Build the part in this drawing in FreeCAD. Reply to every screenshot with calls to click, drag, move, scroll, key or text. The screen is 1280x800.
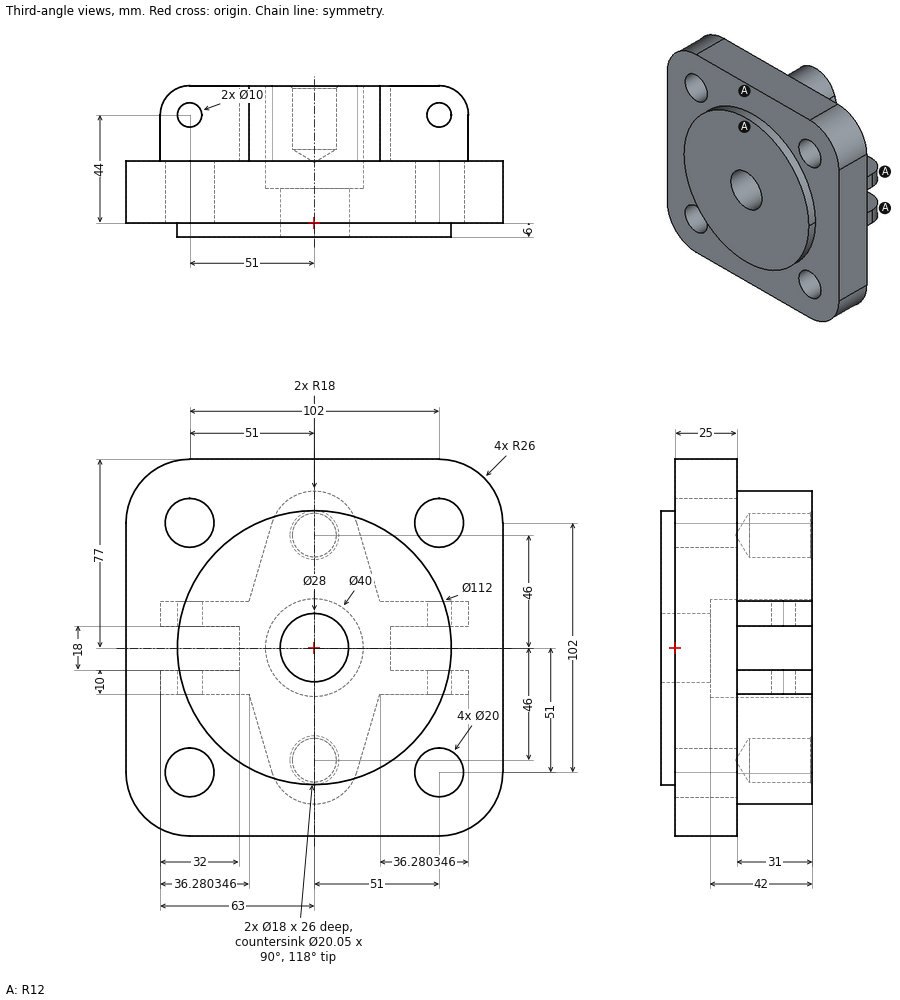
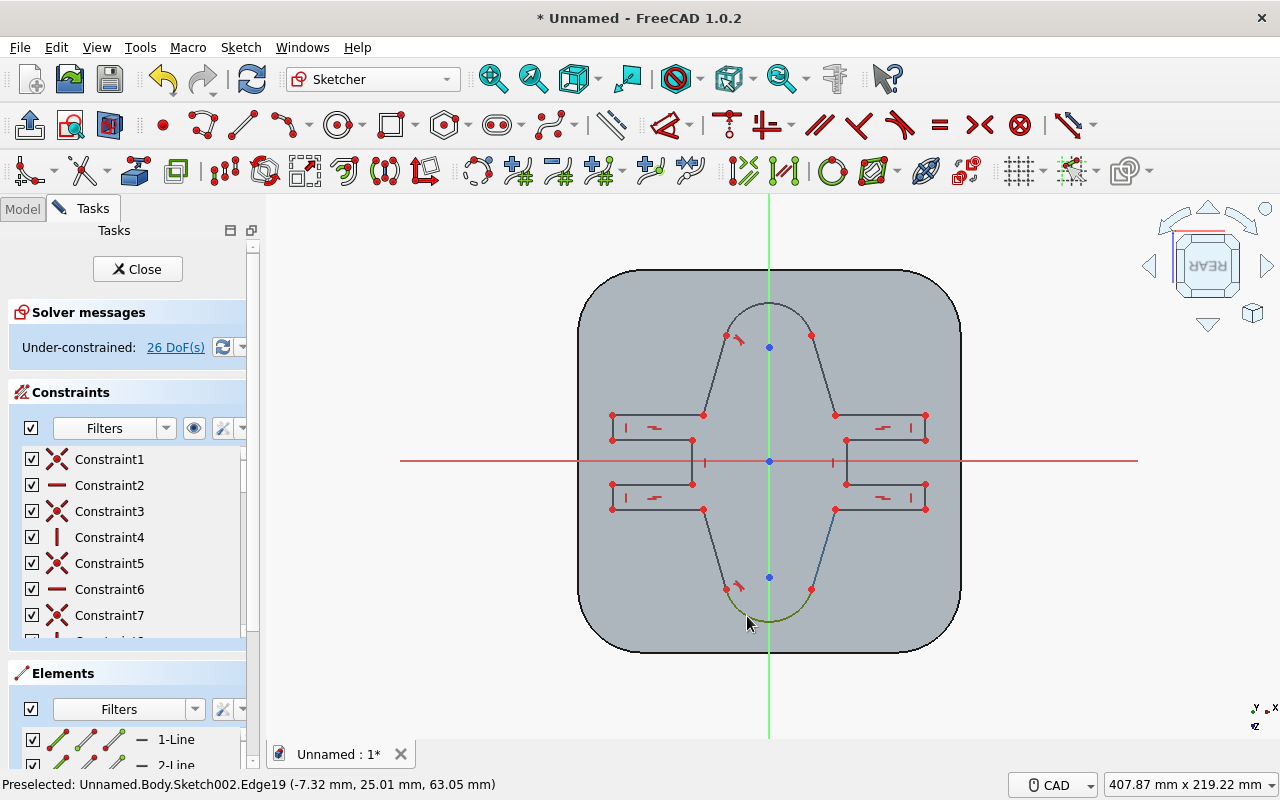
click(900, 126)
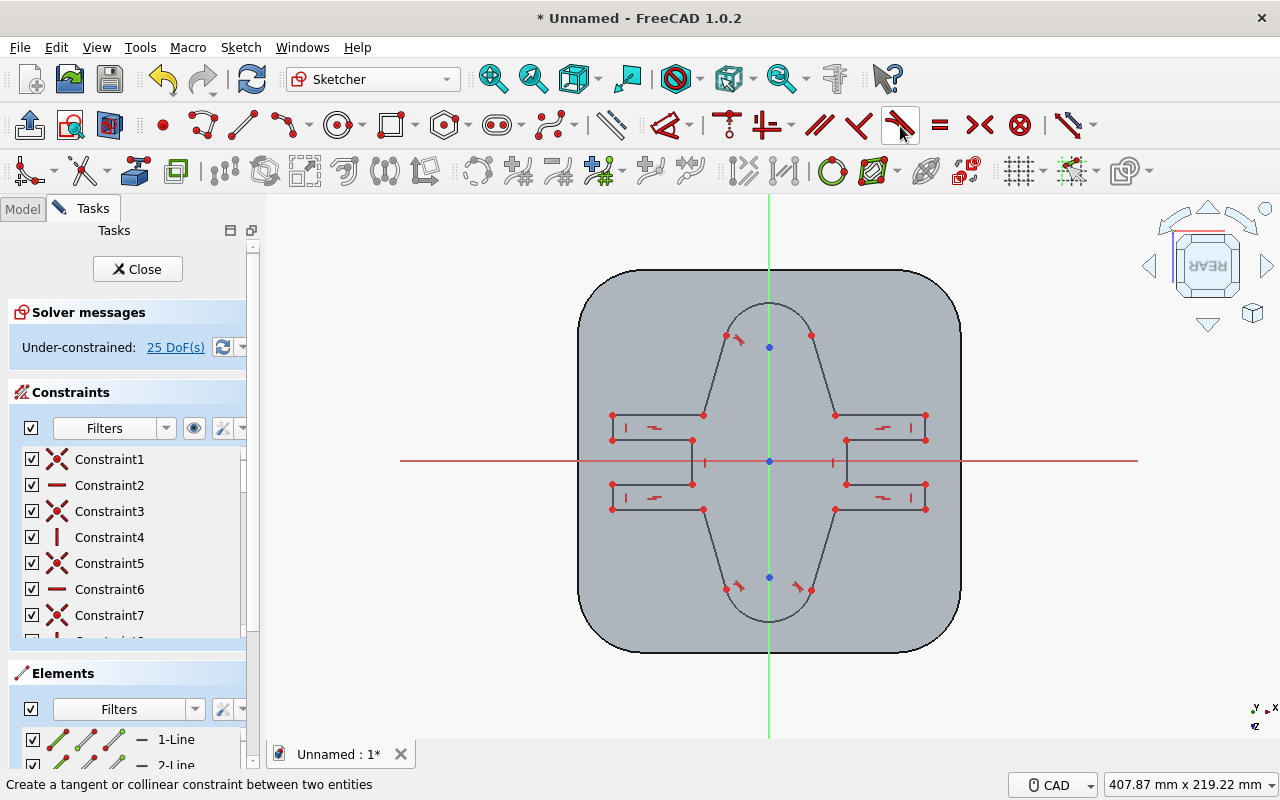
click(829, 391)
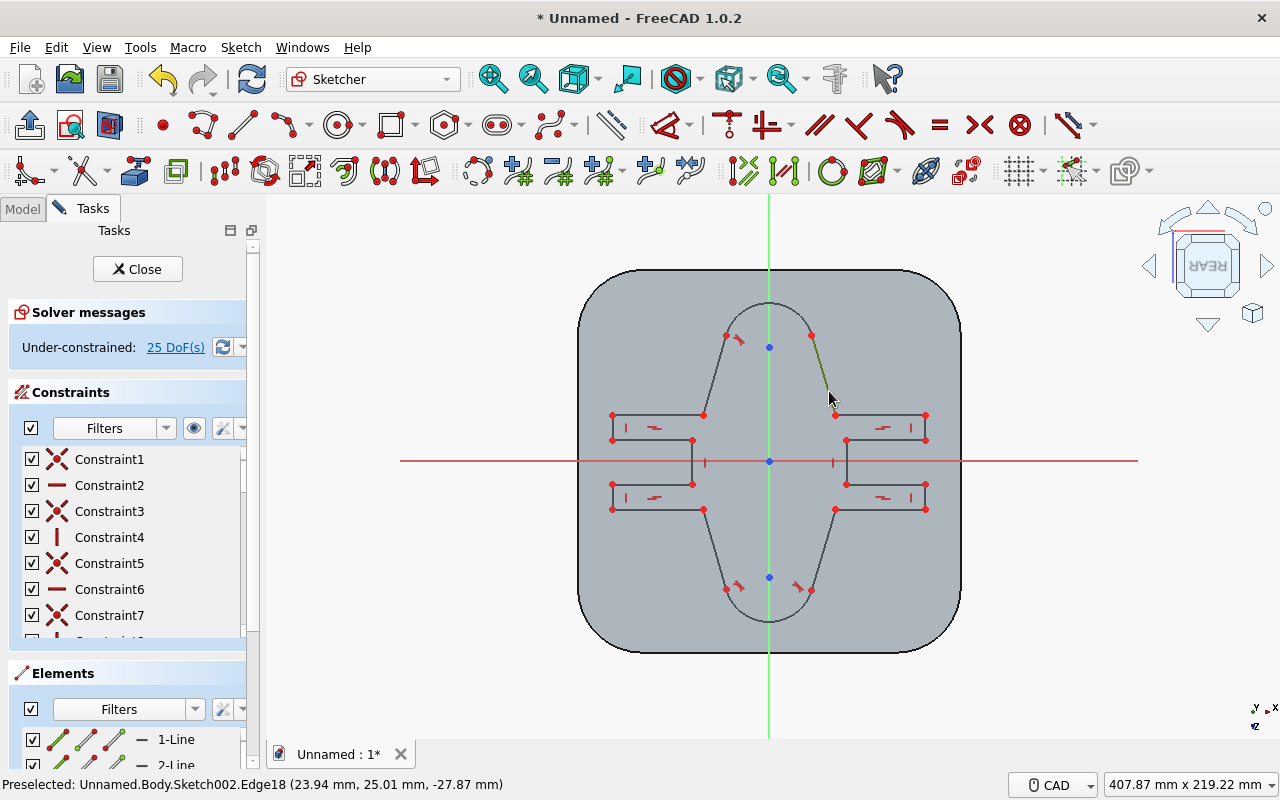
click(791, 309)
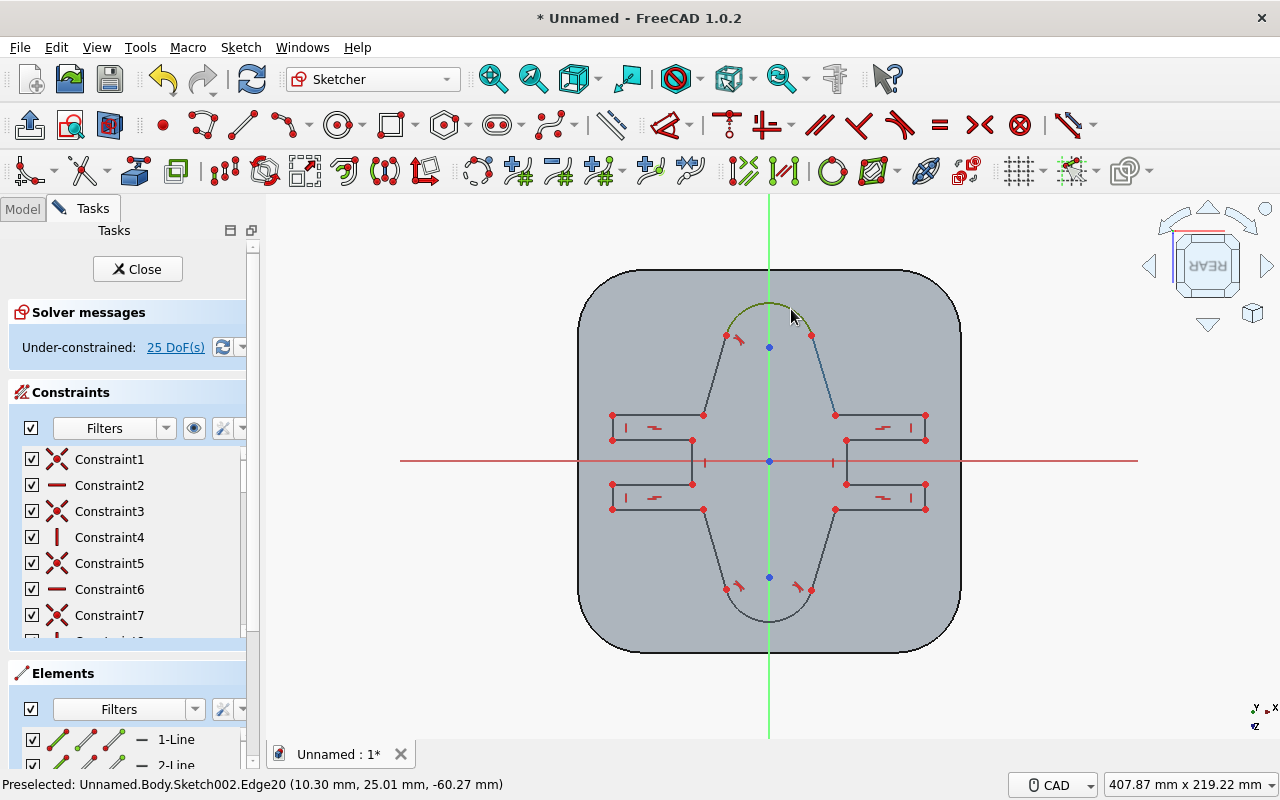
key(t)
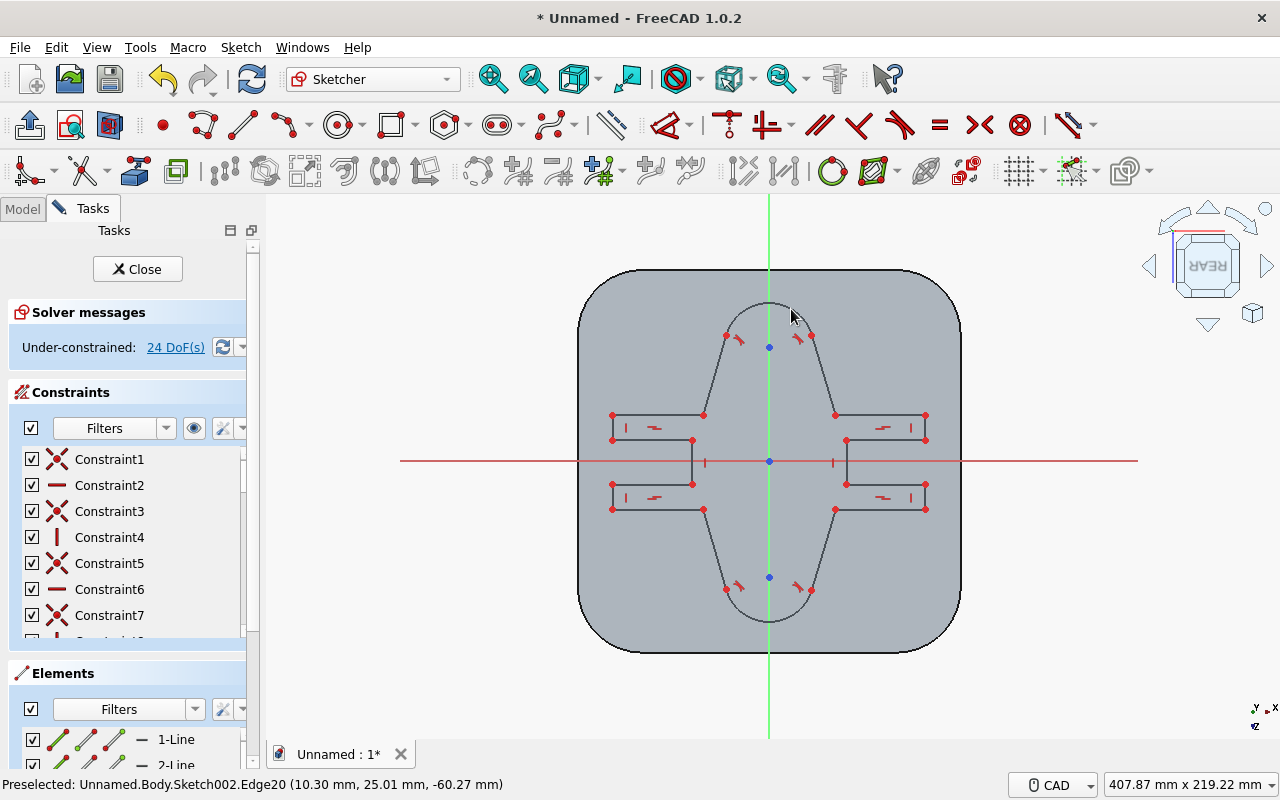
click(747, 616)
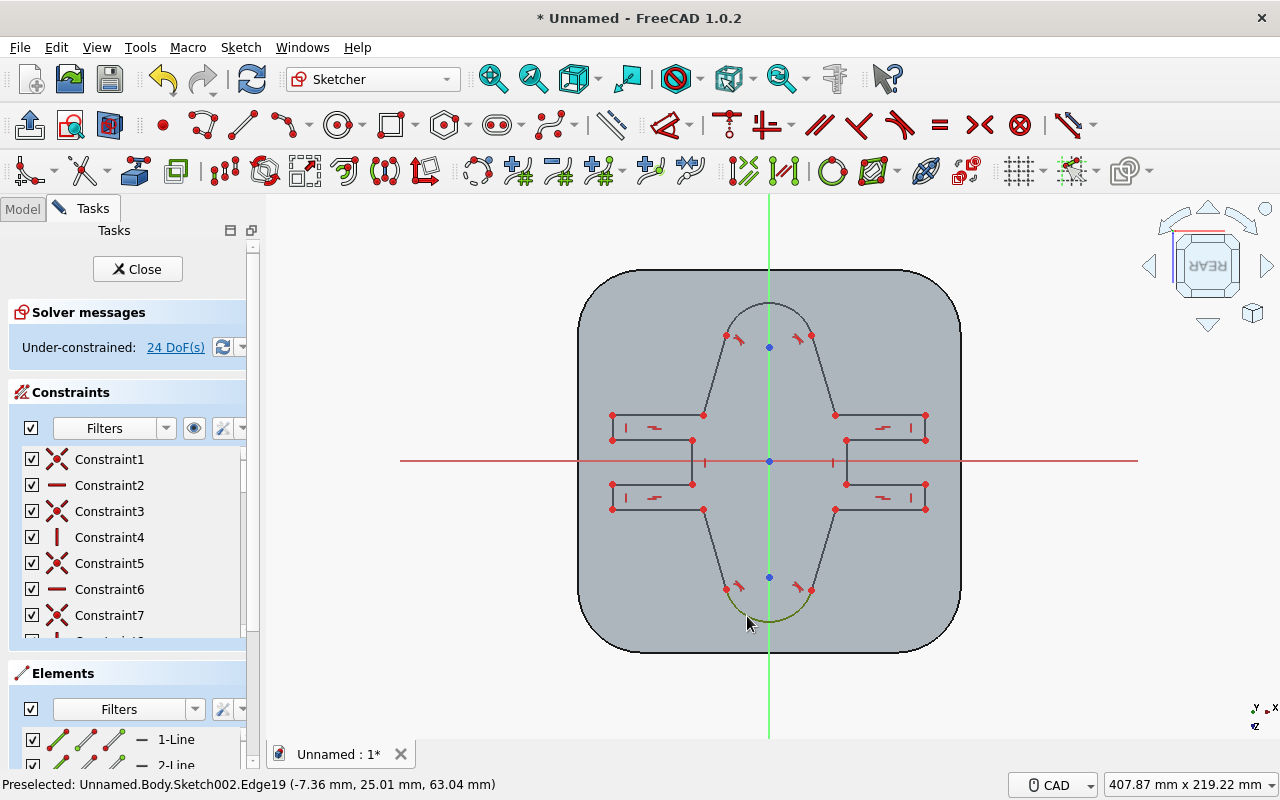
click(791, 309)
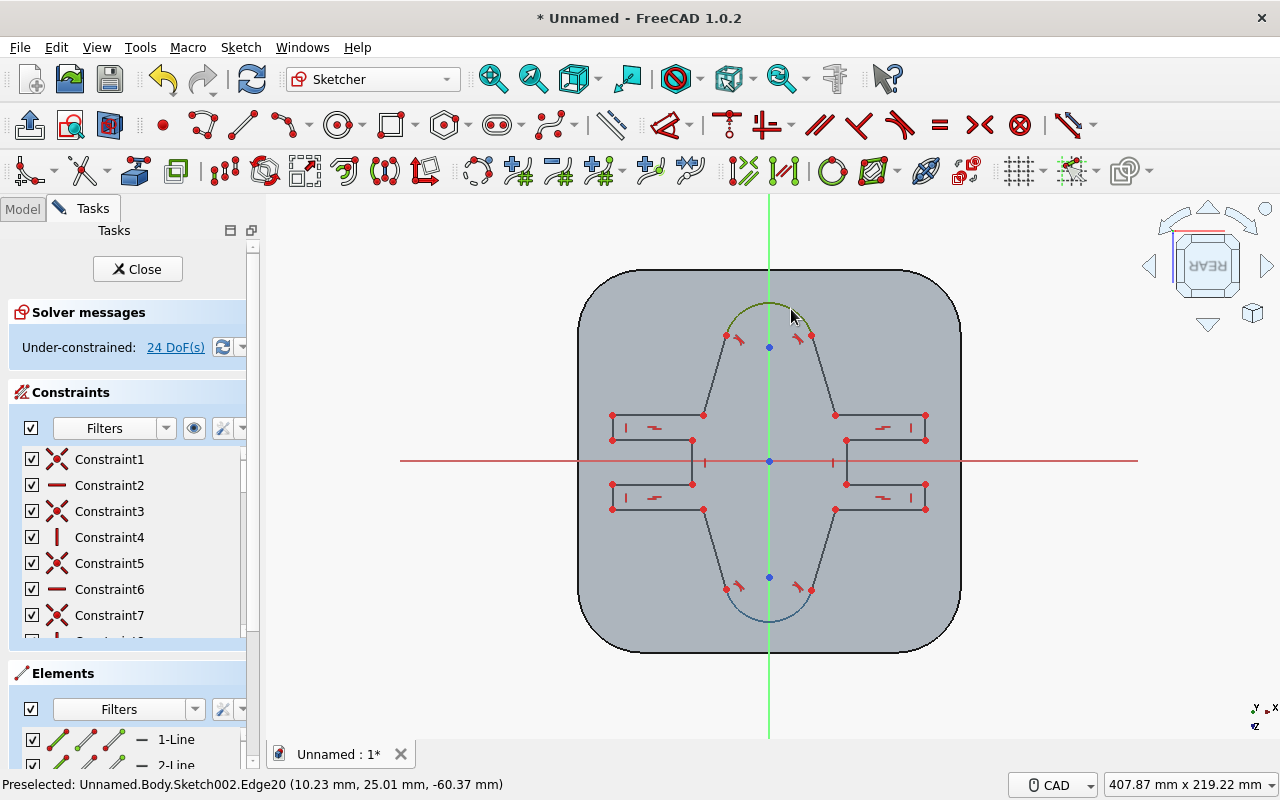
key(e)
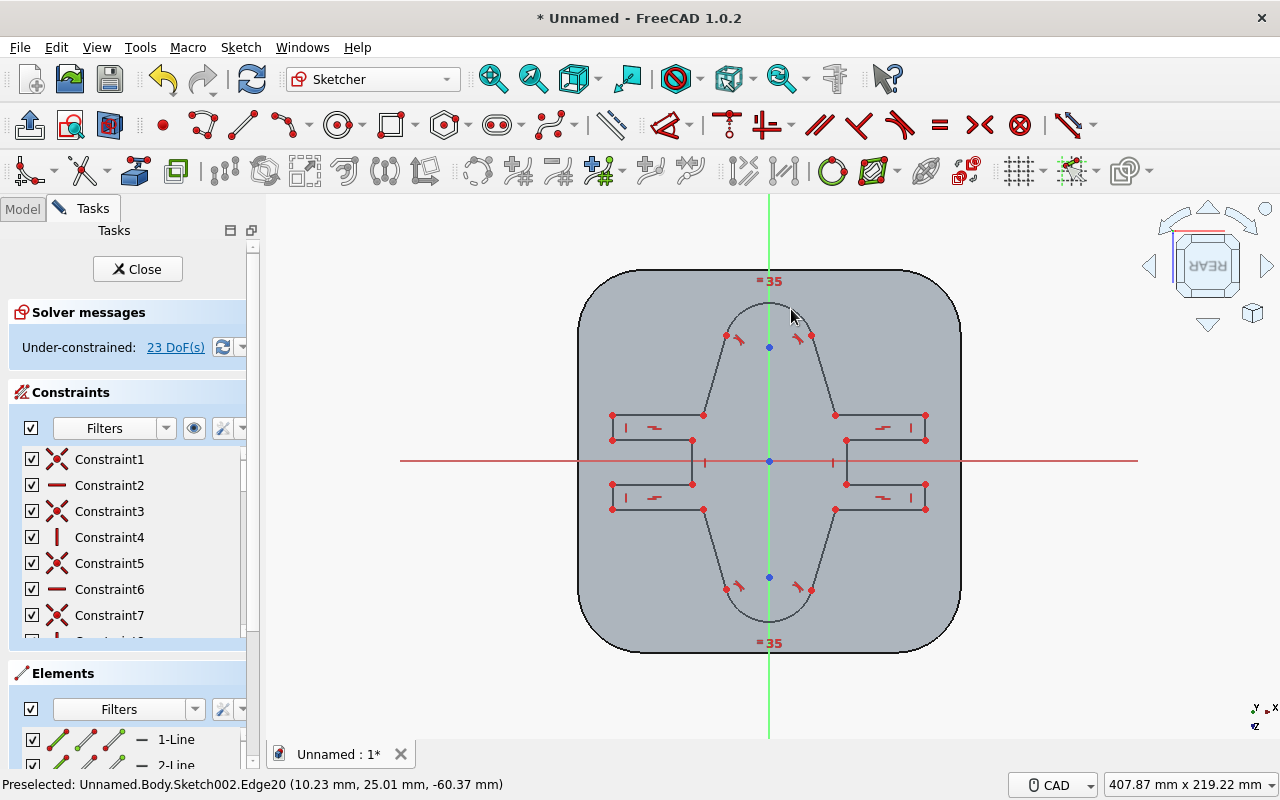
click(769, 577)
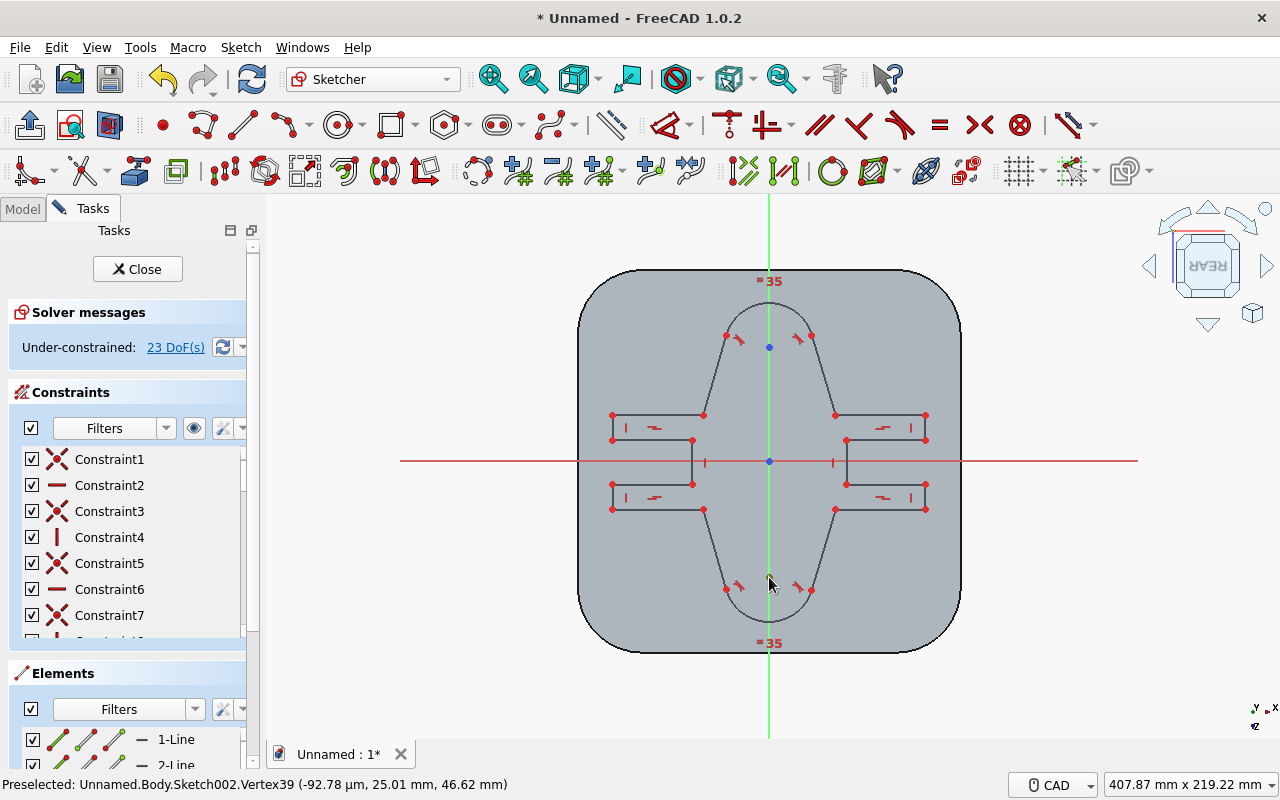
click(769, 676)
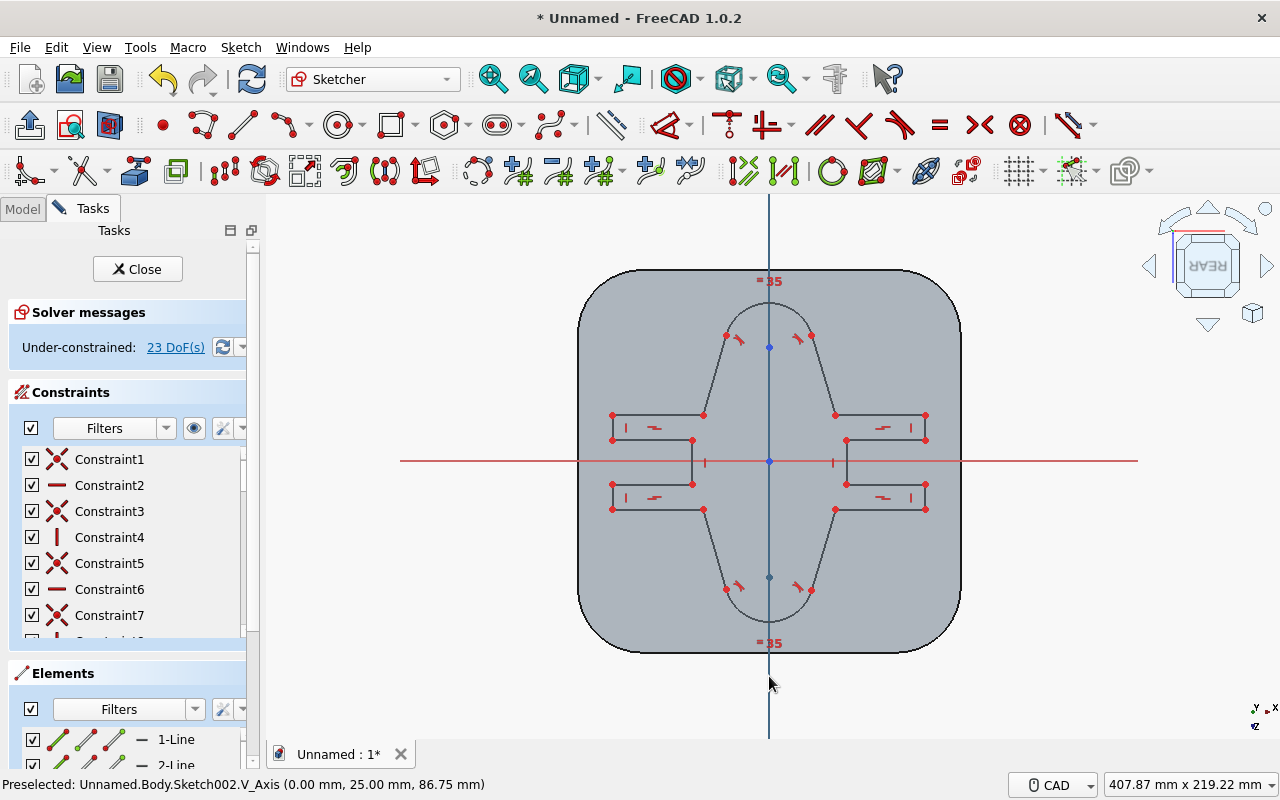
key(c)